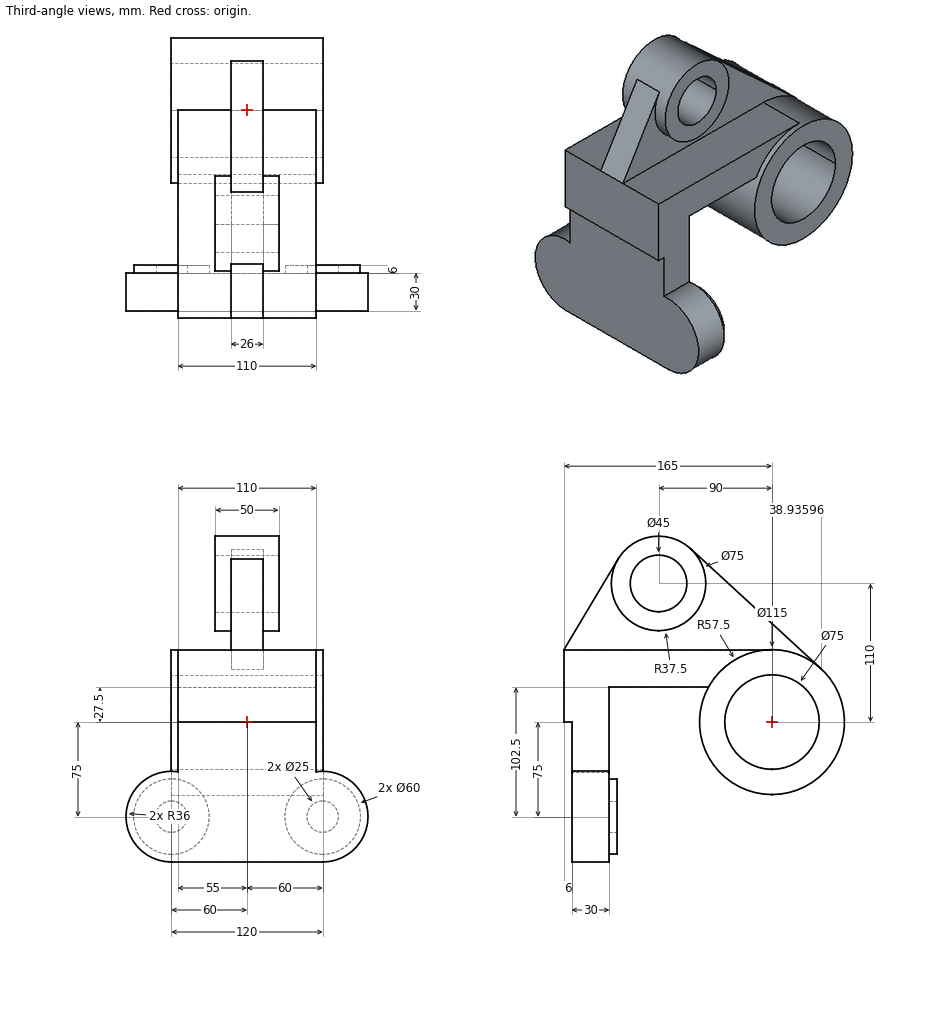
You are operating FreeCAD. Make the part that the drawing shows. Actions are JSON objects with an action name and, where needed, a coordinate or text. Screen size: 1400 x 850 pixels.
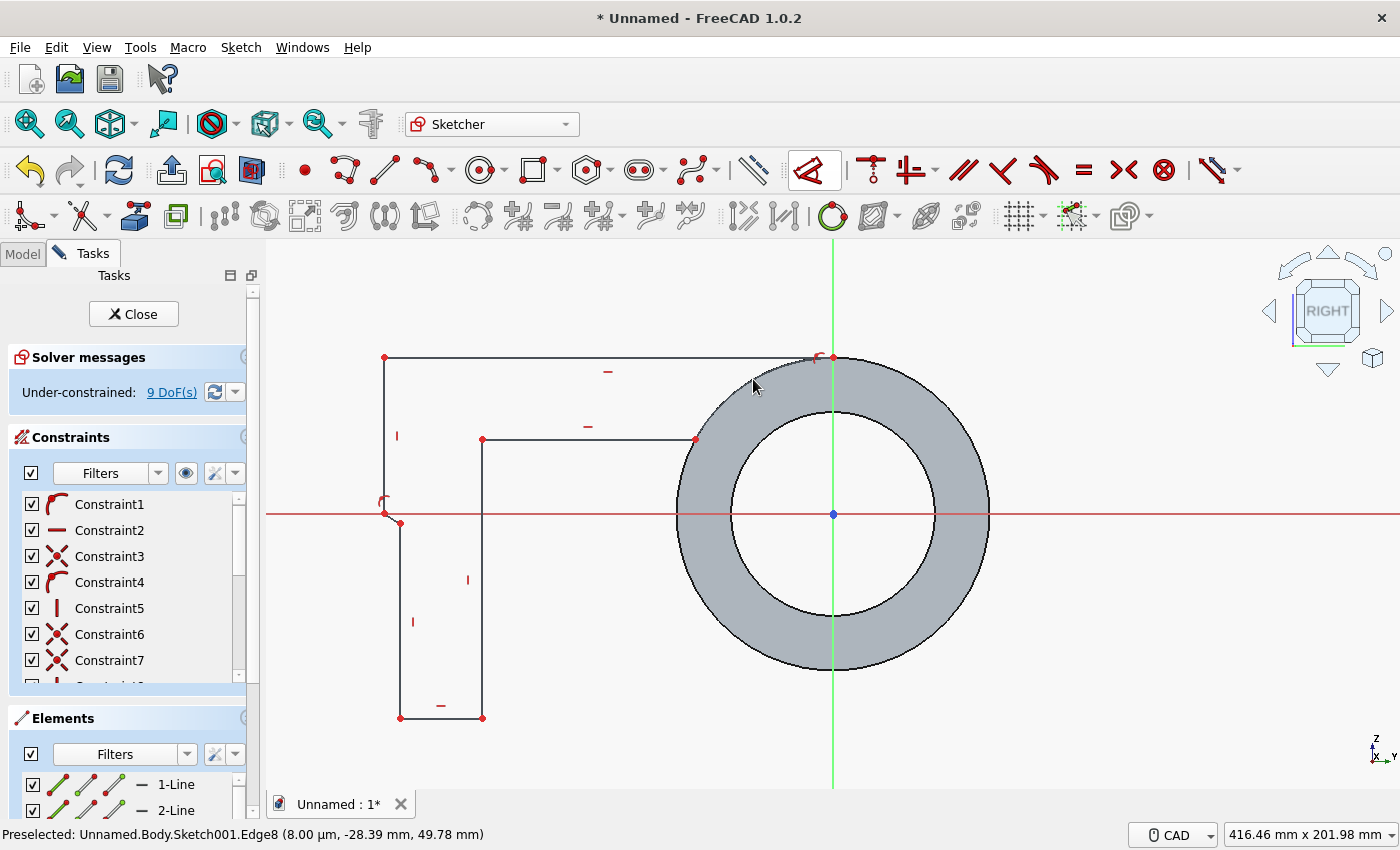
{"action": "scroll", "coordinate": [394, 520], "scroll_direction": "up", "scroll_amount": 5}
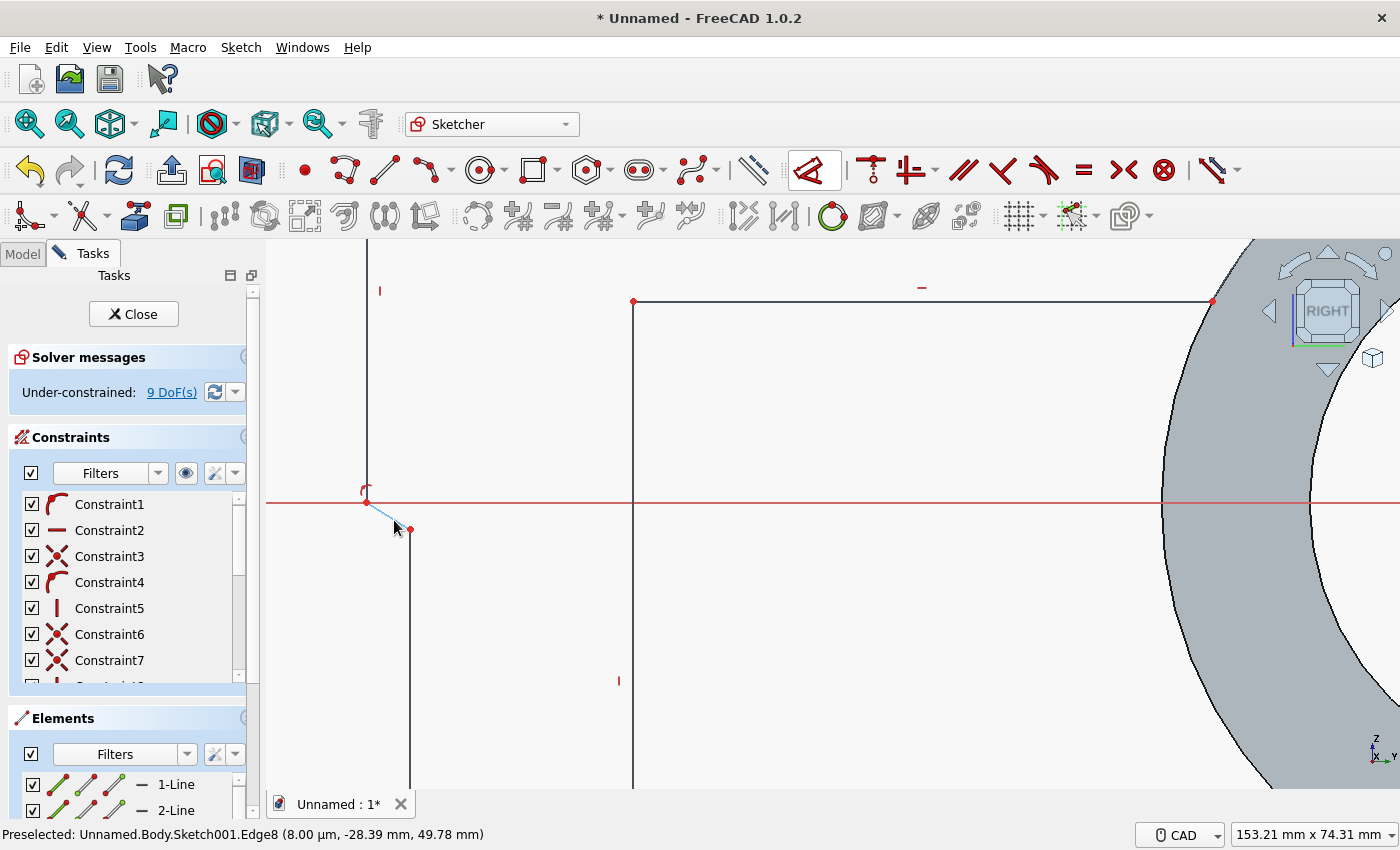
{"action": "left_click", "coordinate": [393, 519]}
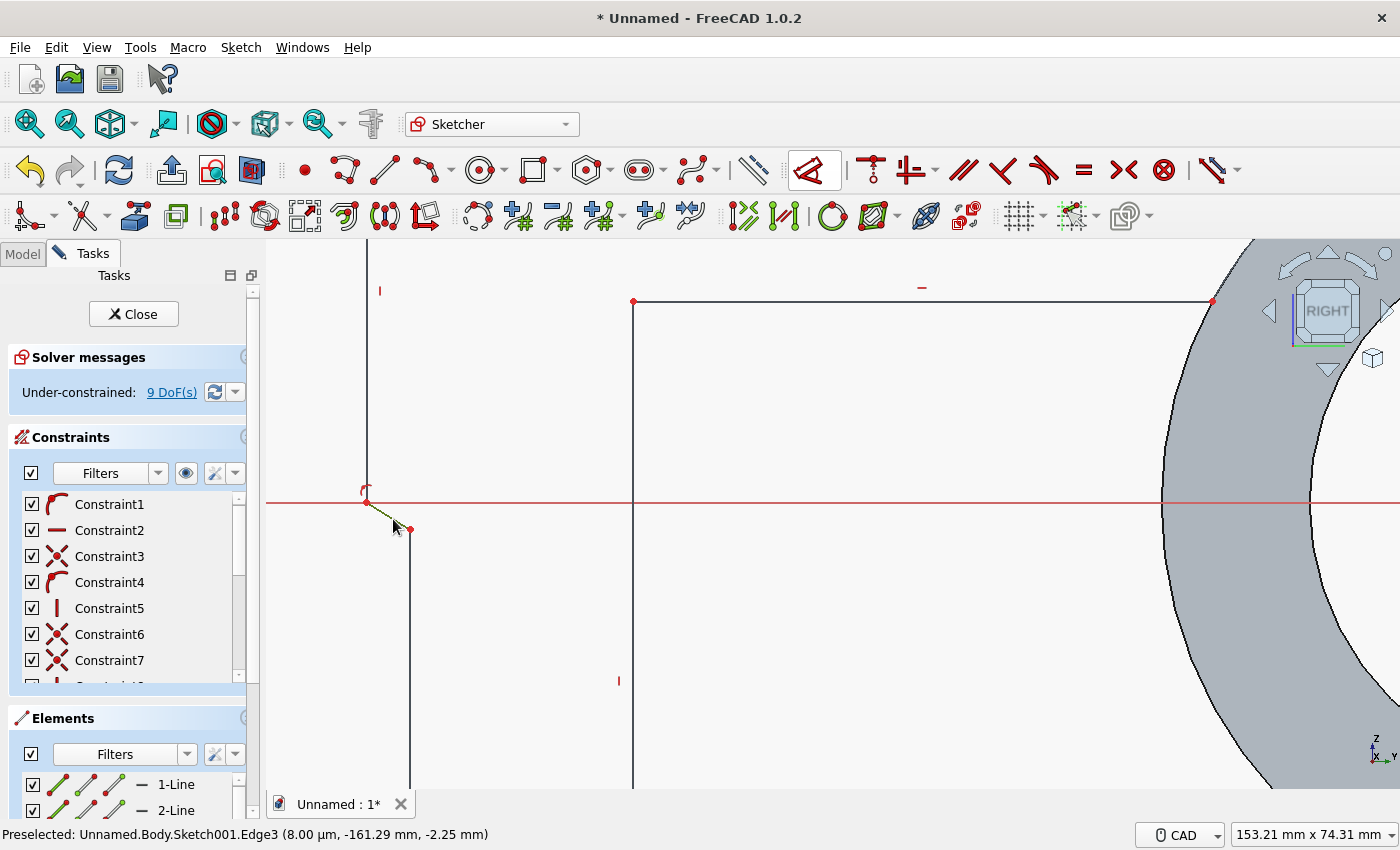
{"action": "left_click", "coordinate": [938, 170]}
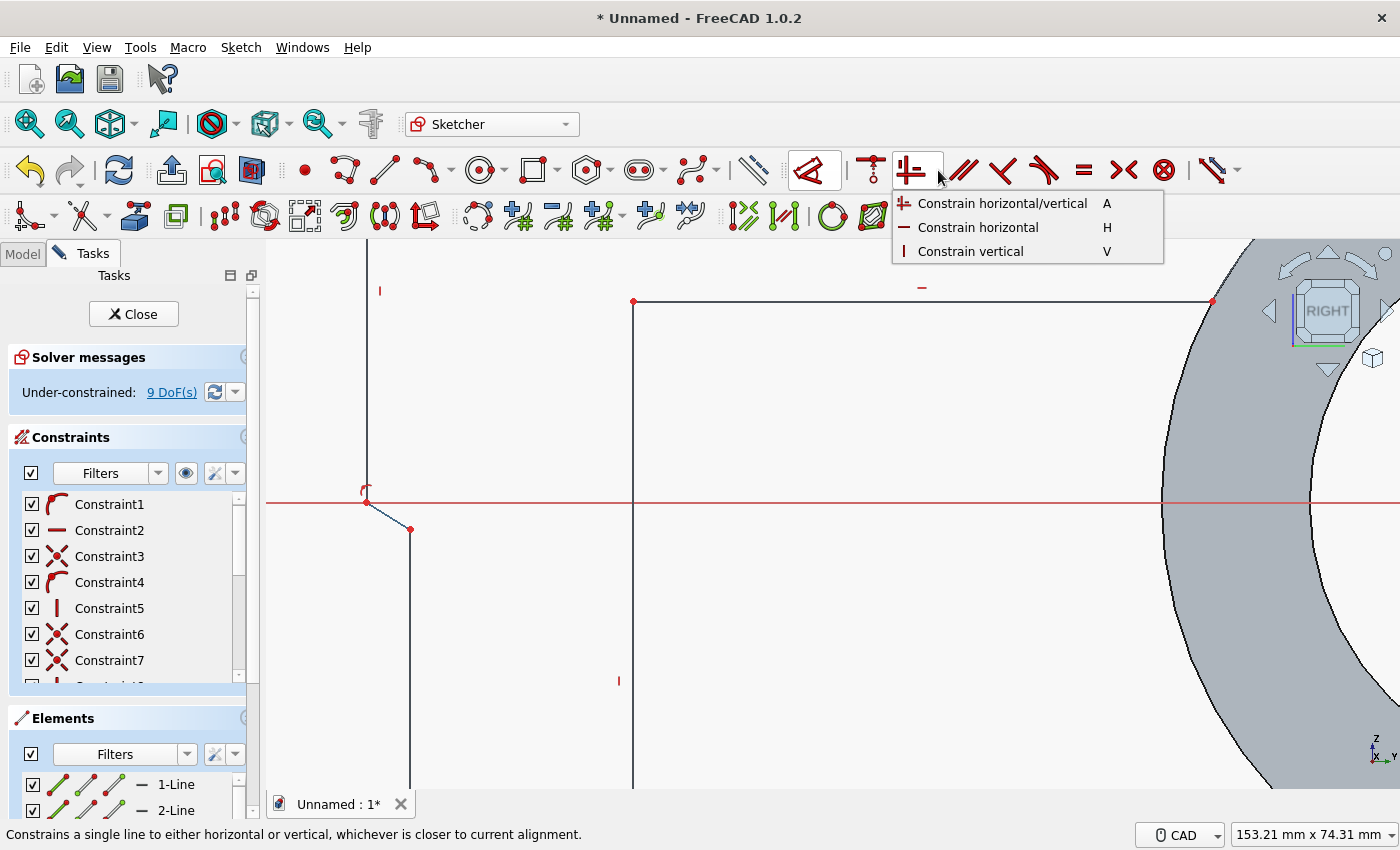
{"action": "left_click", "coordinate": [1028, 227]}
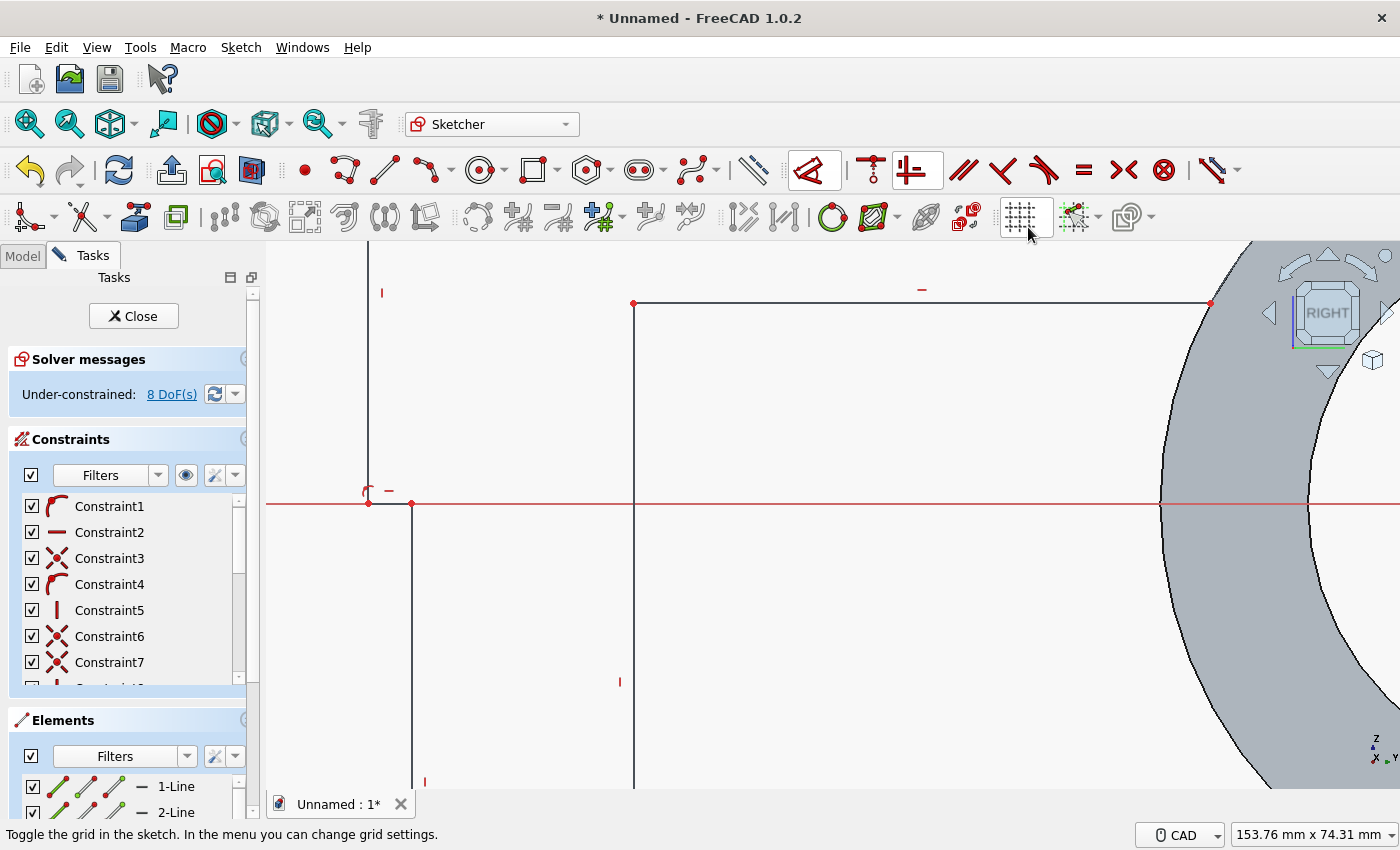
{"action": "scroll", "coordinate": [641, 484], "scroll_direction": "down", "scroll_amount": 5}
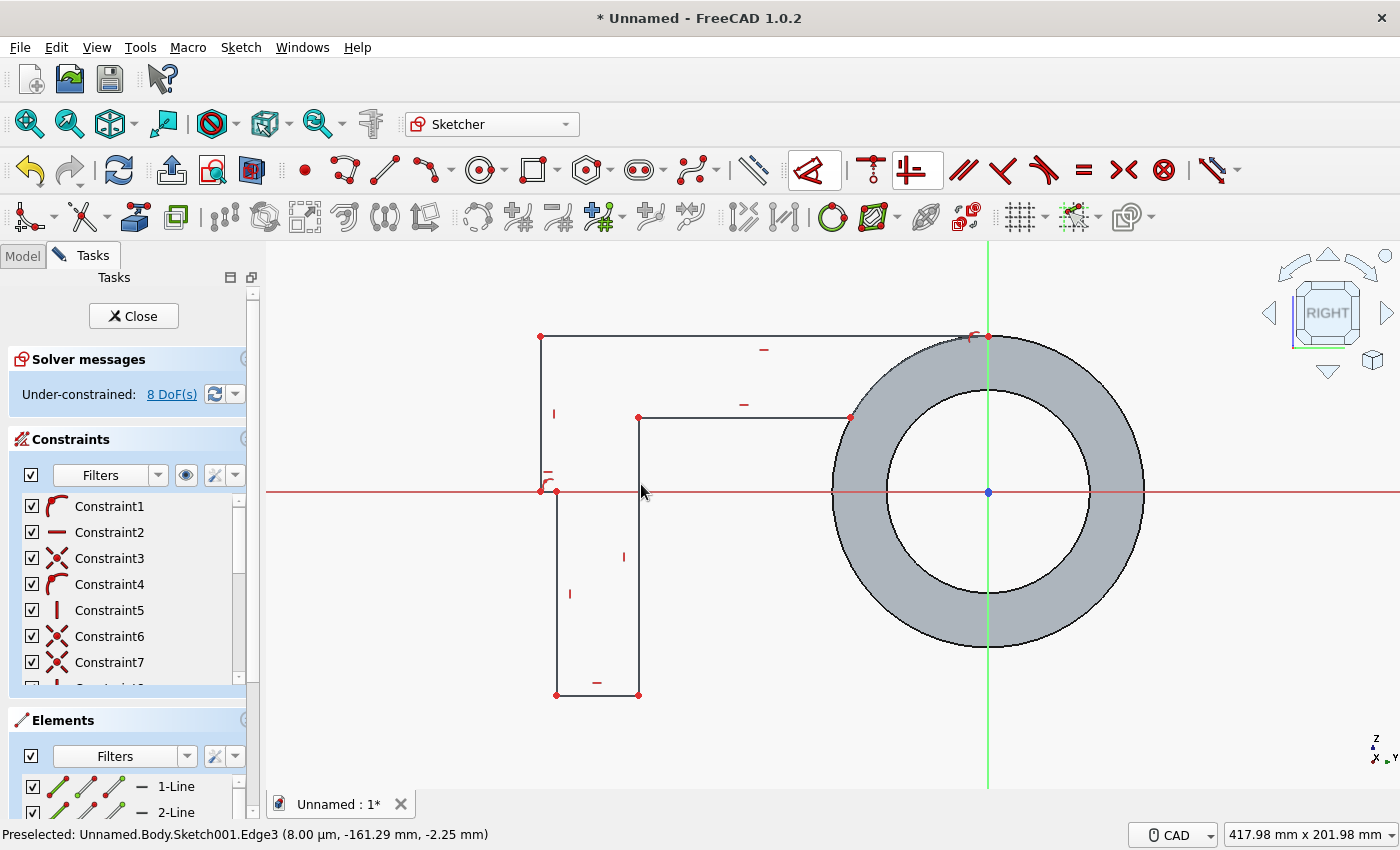
{"action": "left_click_drag", "start_coordinate": [978, 482], "coordinate": [999, 503]}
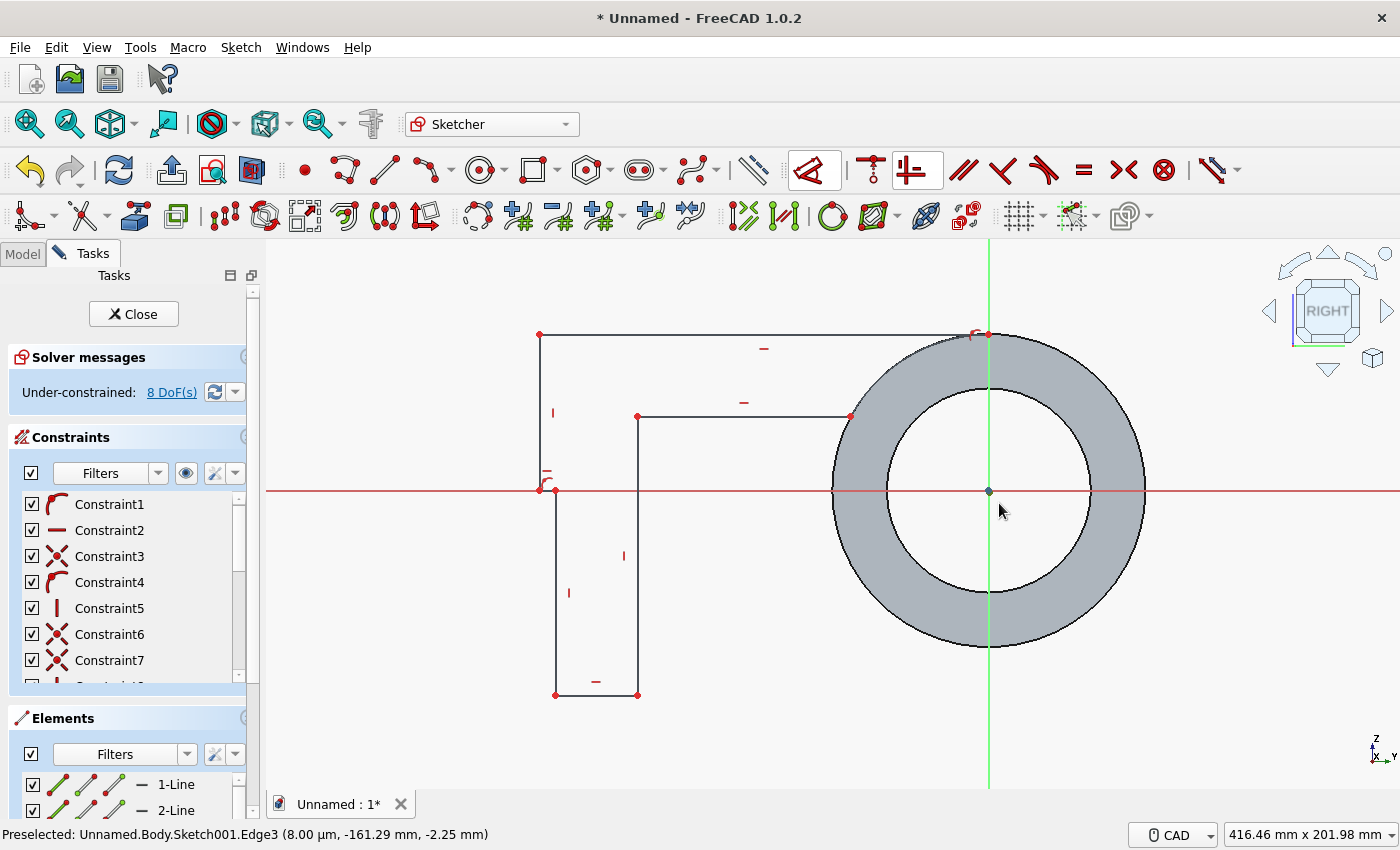
{"action": "left_click", "coordinate": [872, 170]}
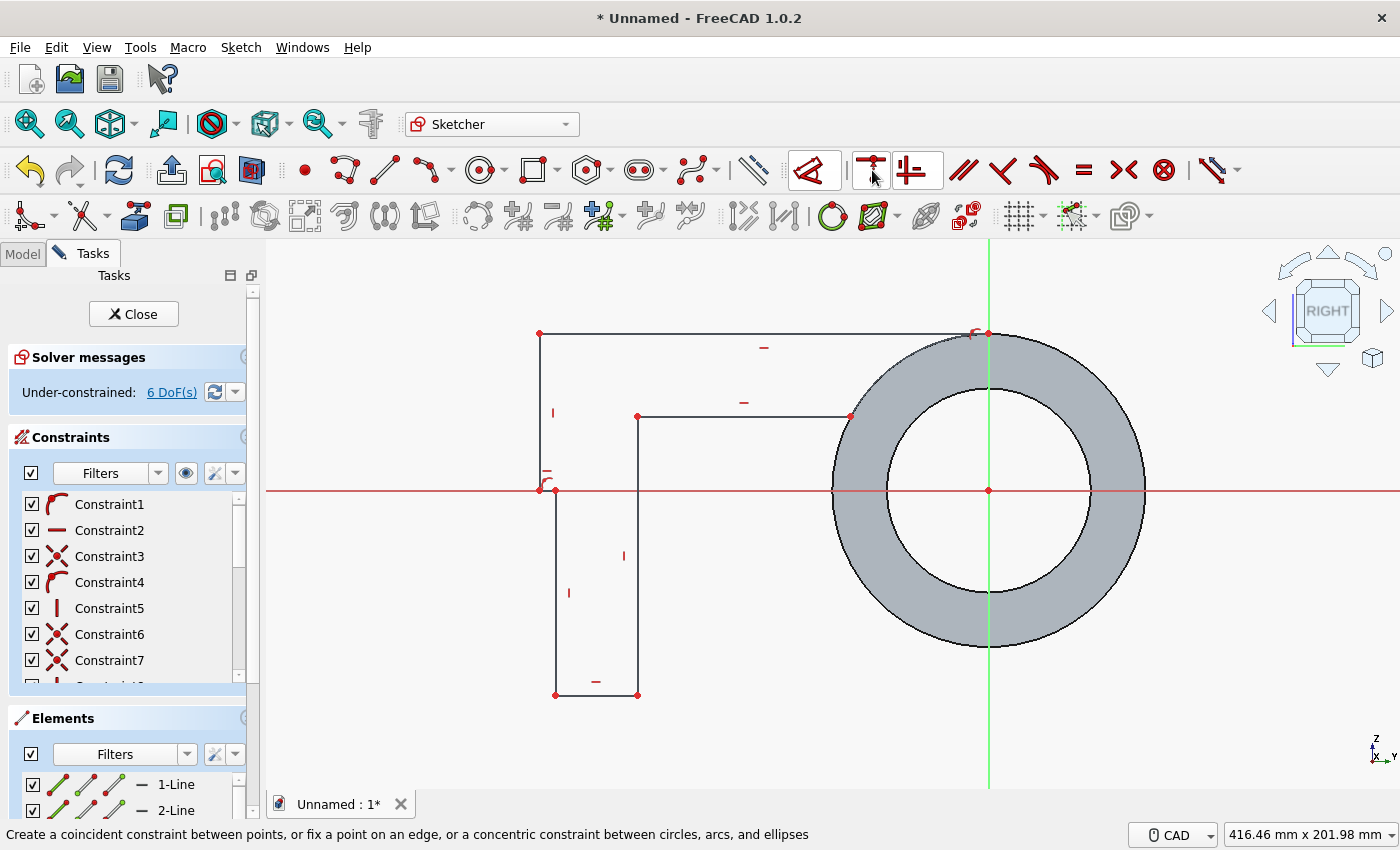
{"action": "left_click", "coordinate": [808, 170]}